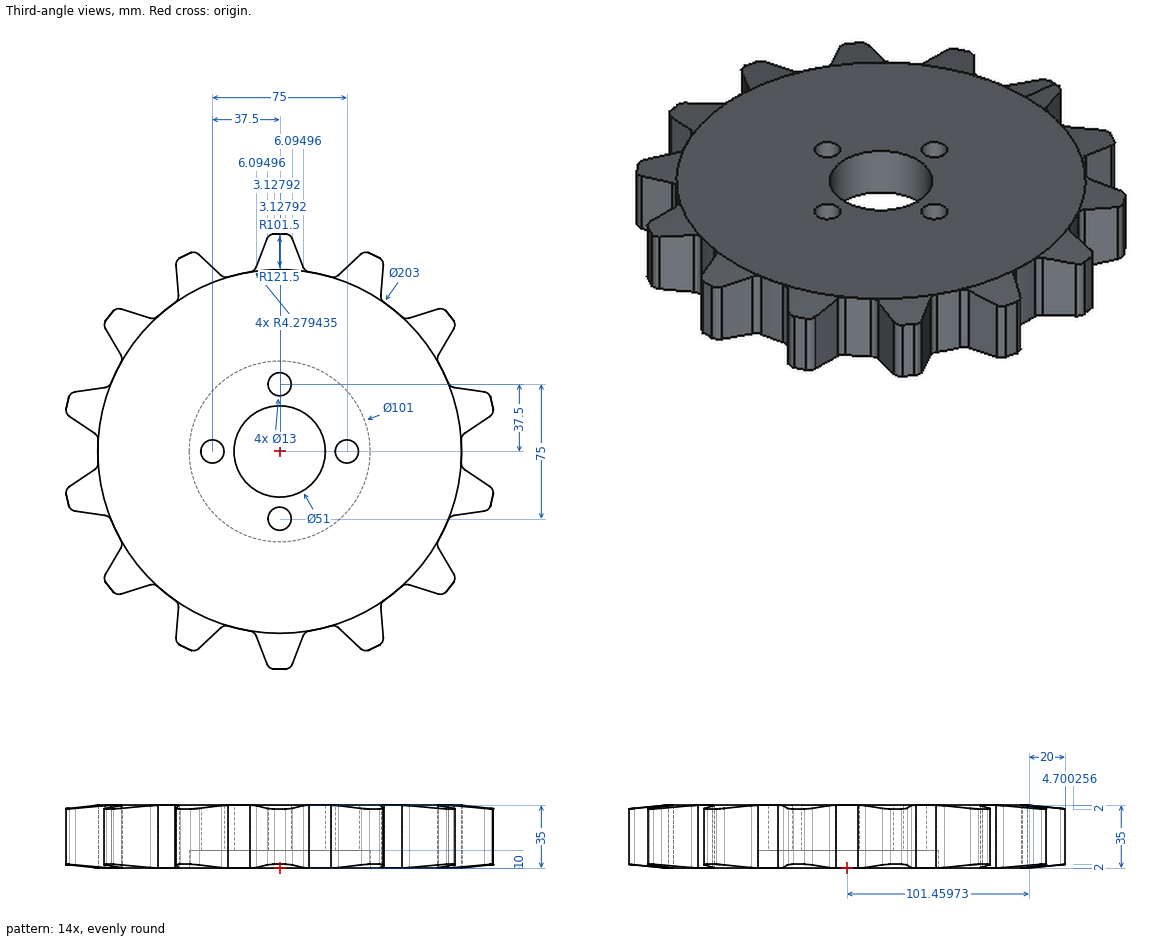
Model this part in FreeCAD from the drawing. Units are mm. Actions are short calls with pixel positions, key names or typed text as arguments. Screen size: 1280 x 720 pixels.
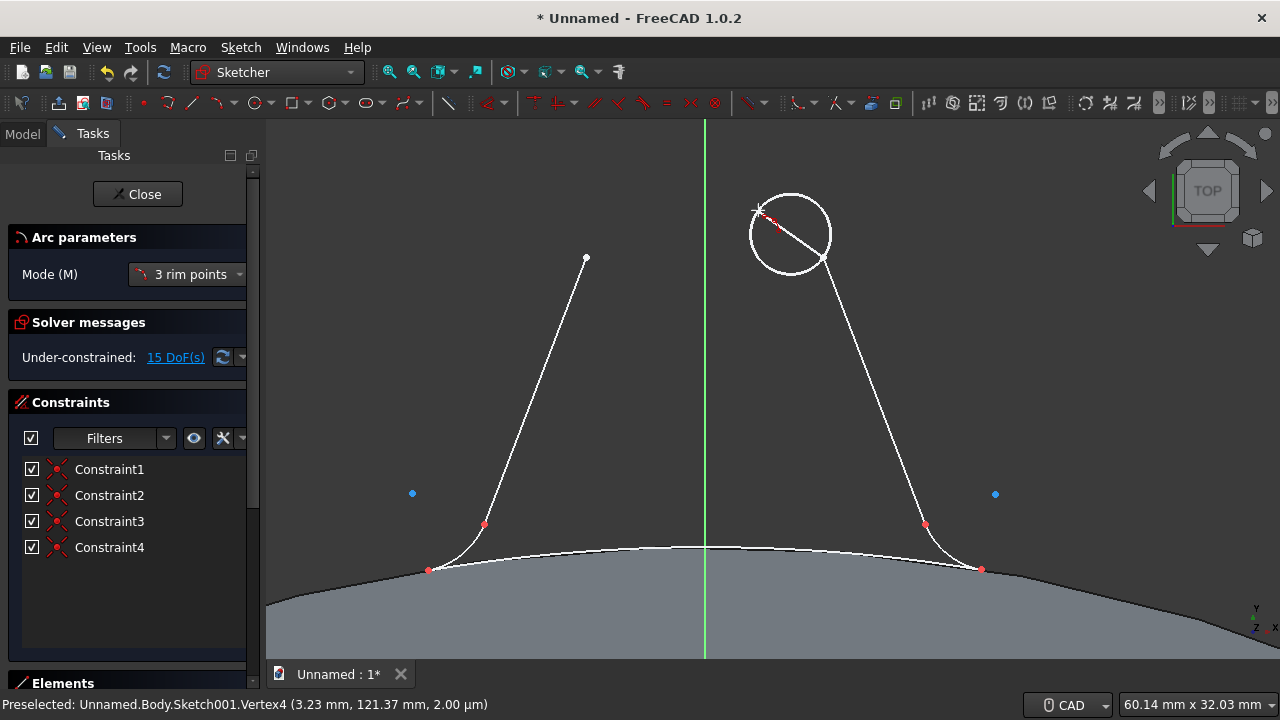
scroll(797, 223, up, 2)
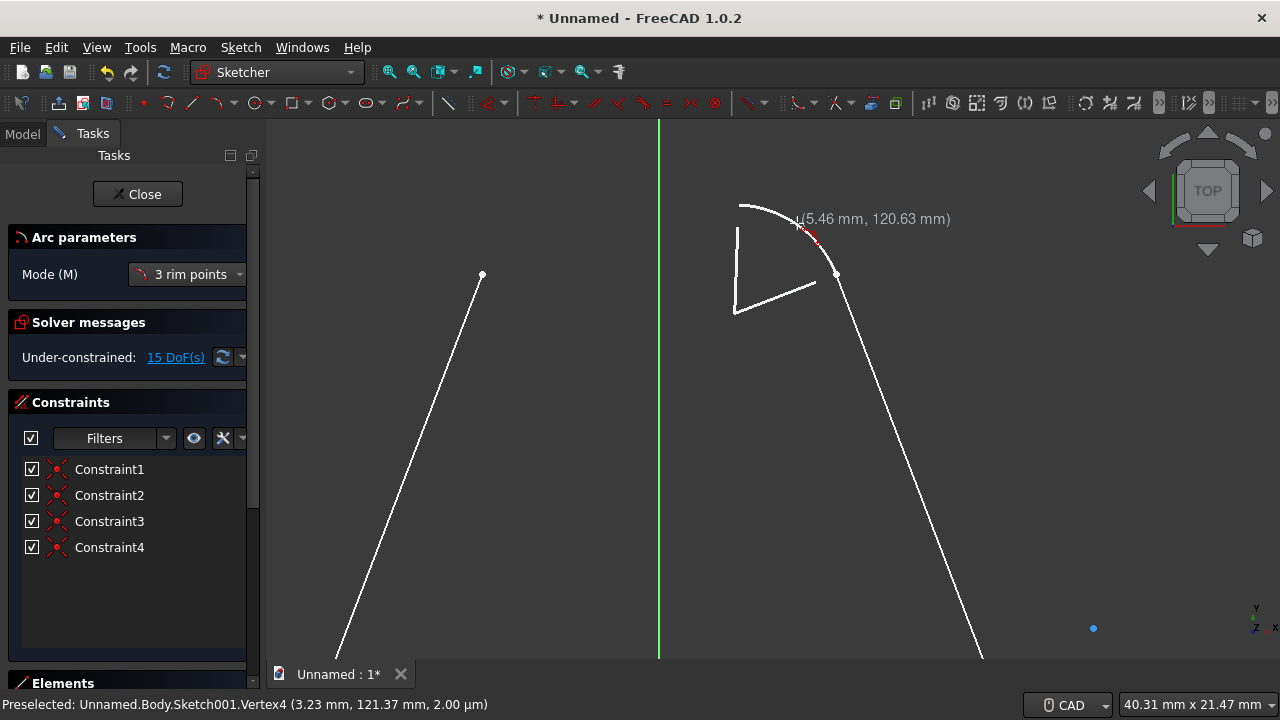
click(797, 223)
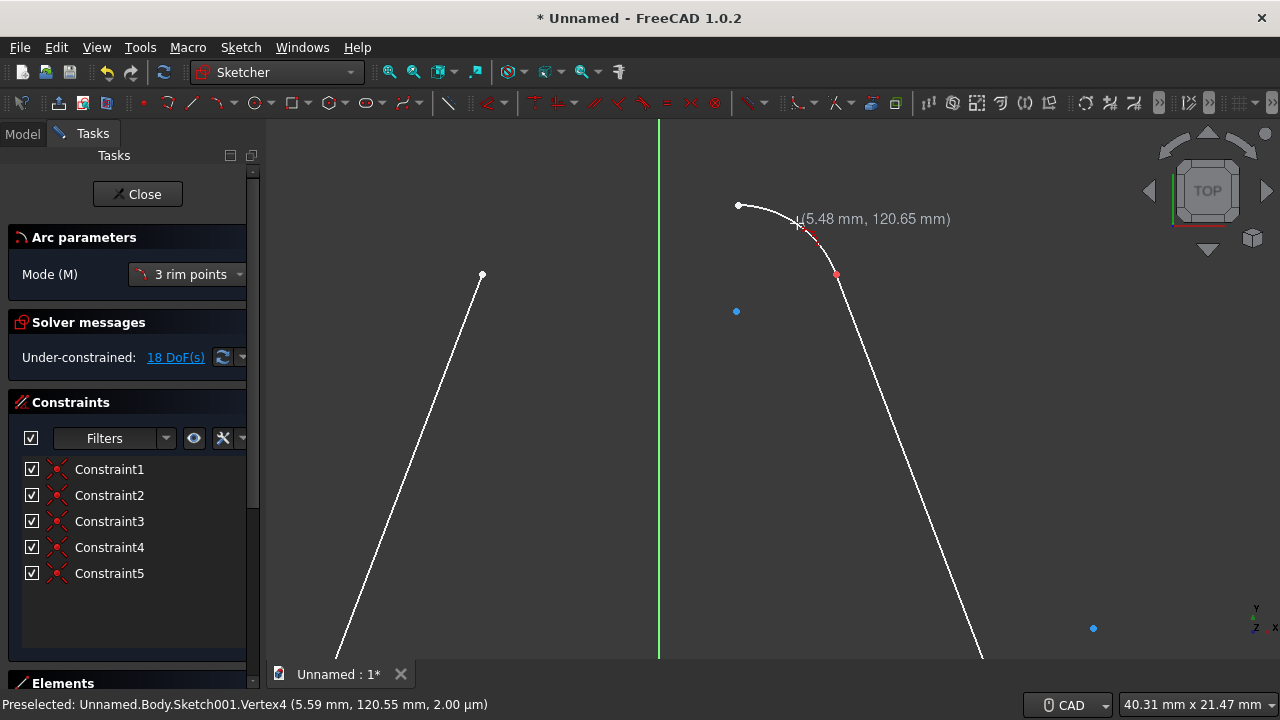
click(739, 205)
click(581, 204)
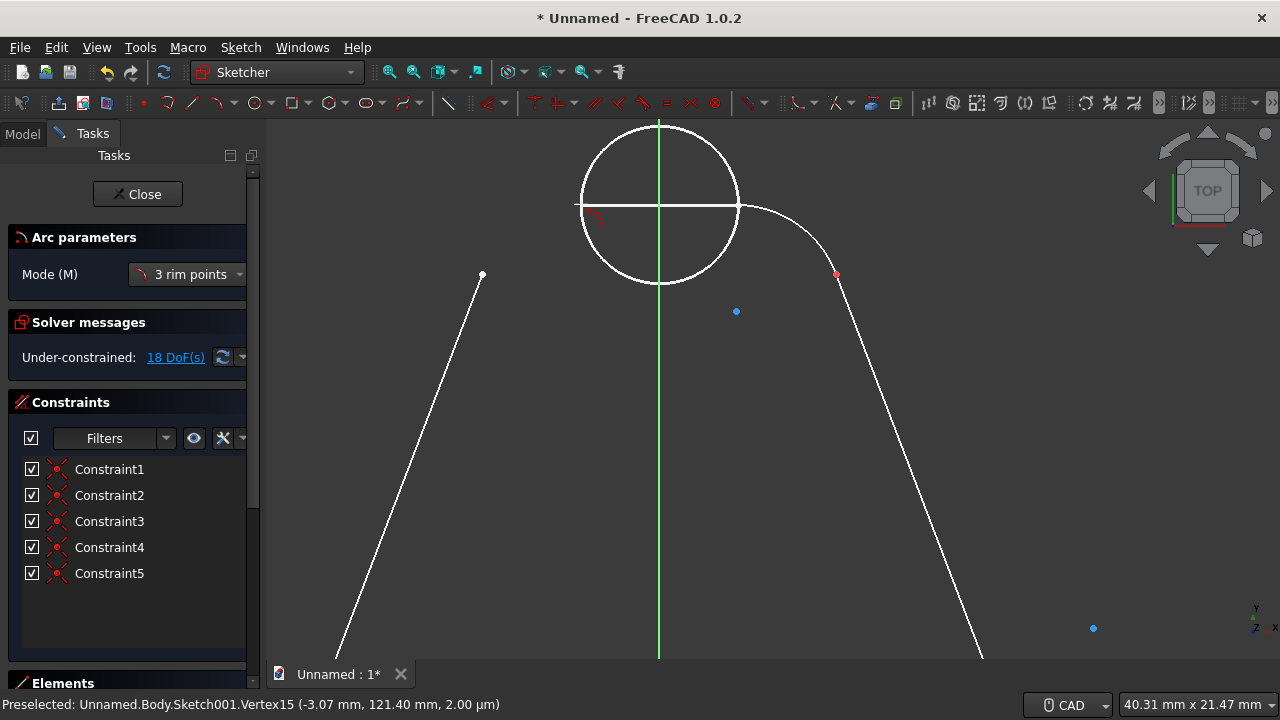
scroll(675, 203, up, 14)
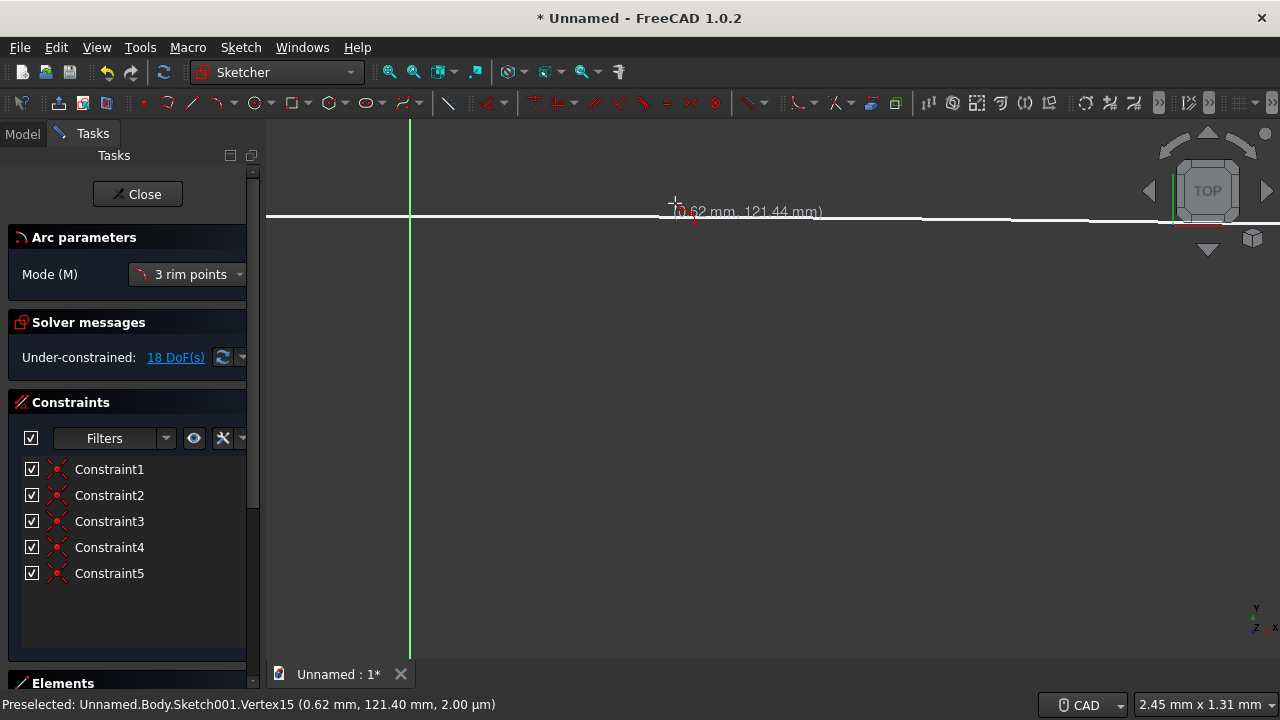
click(669, 194)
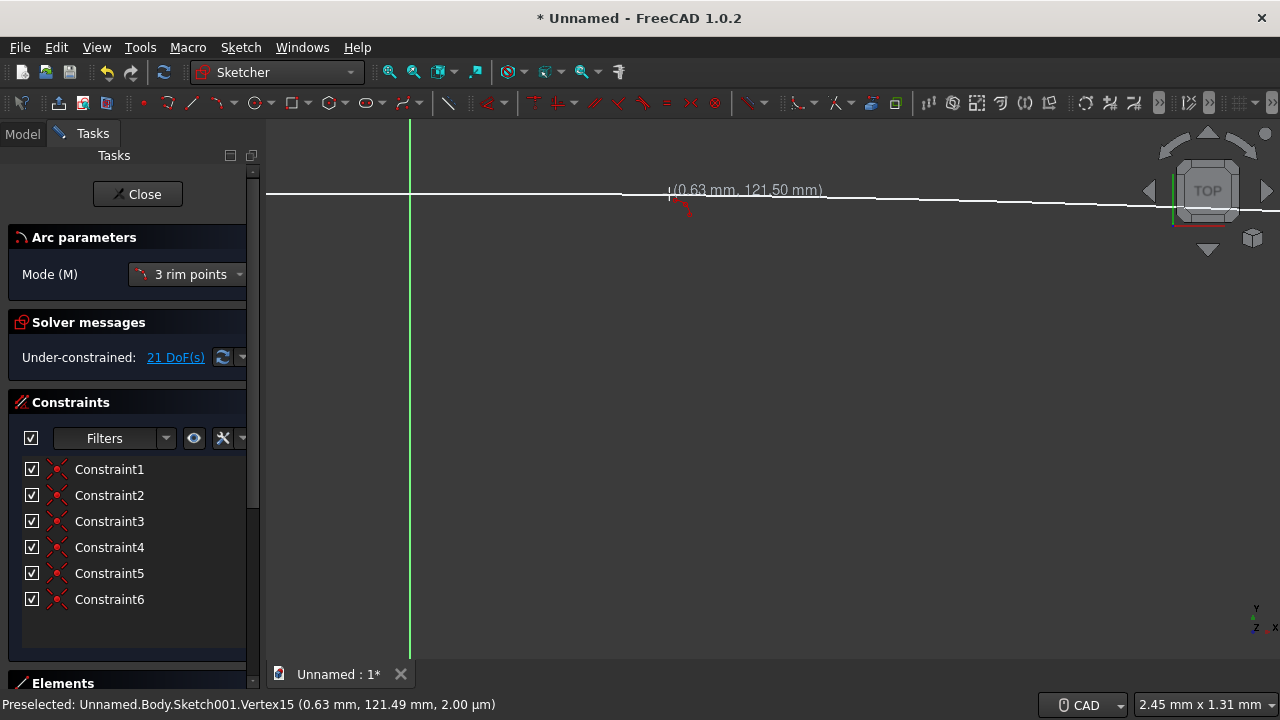
scroll(717, 210, down, 16)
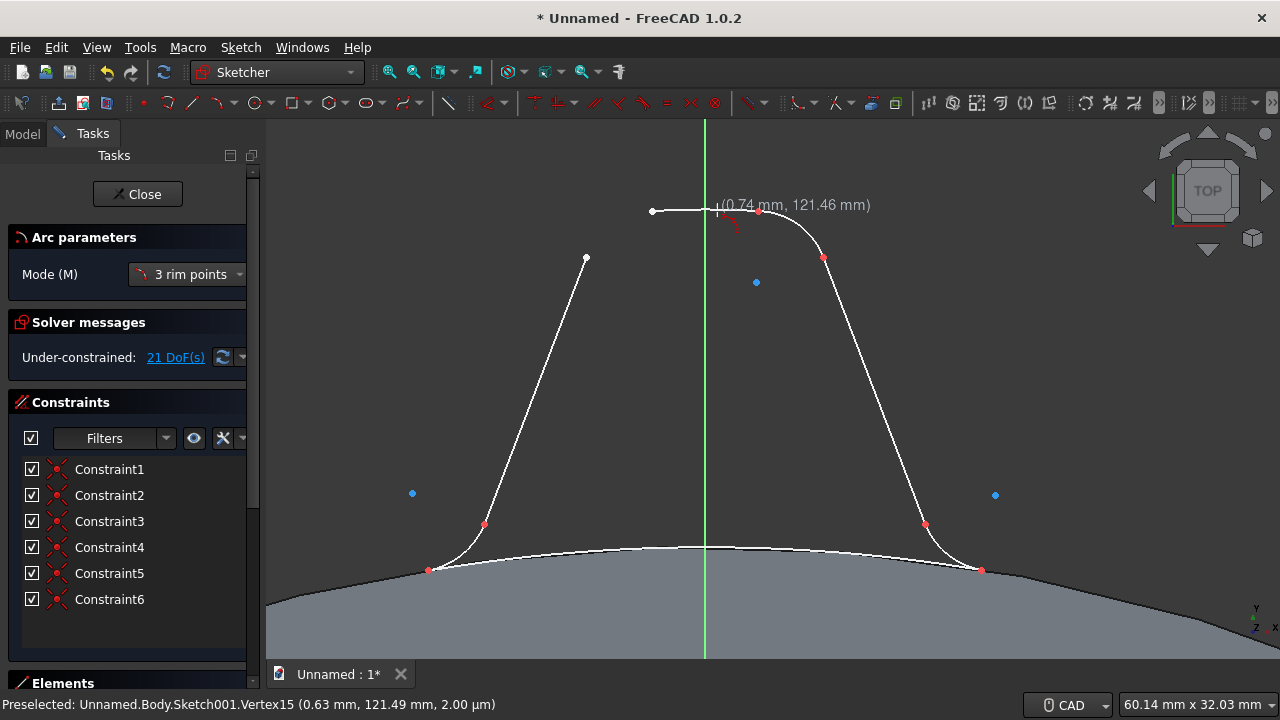
click(652, 211)
click(586, 258)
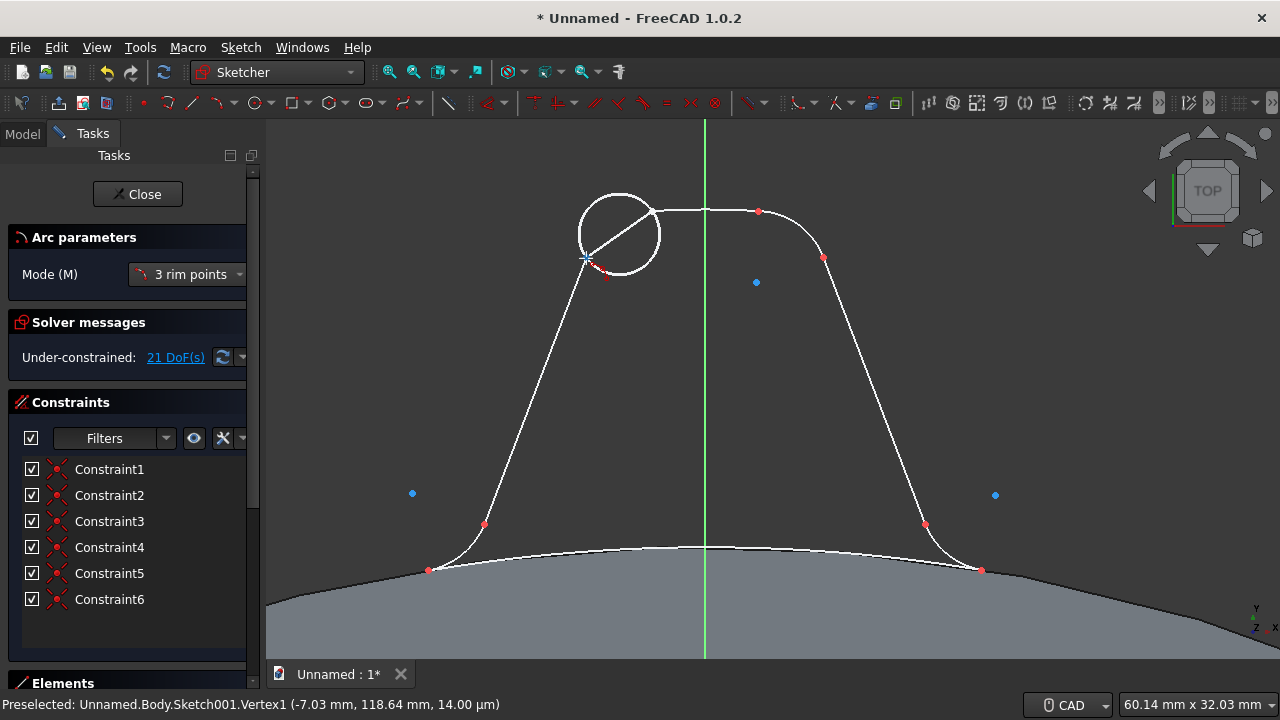
scroll(612, 223, up, 2)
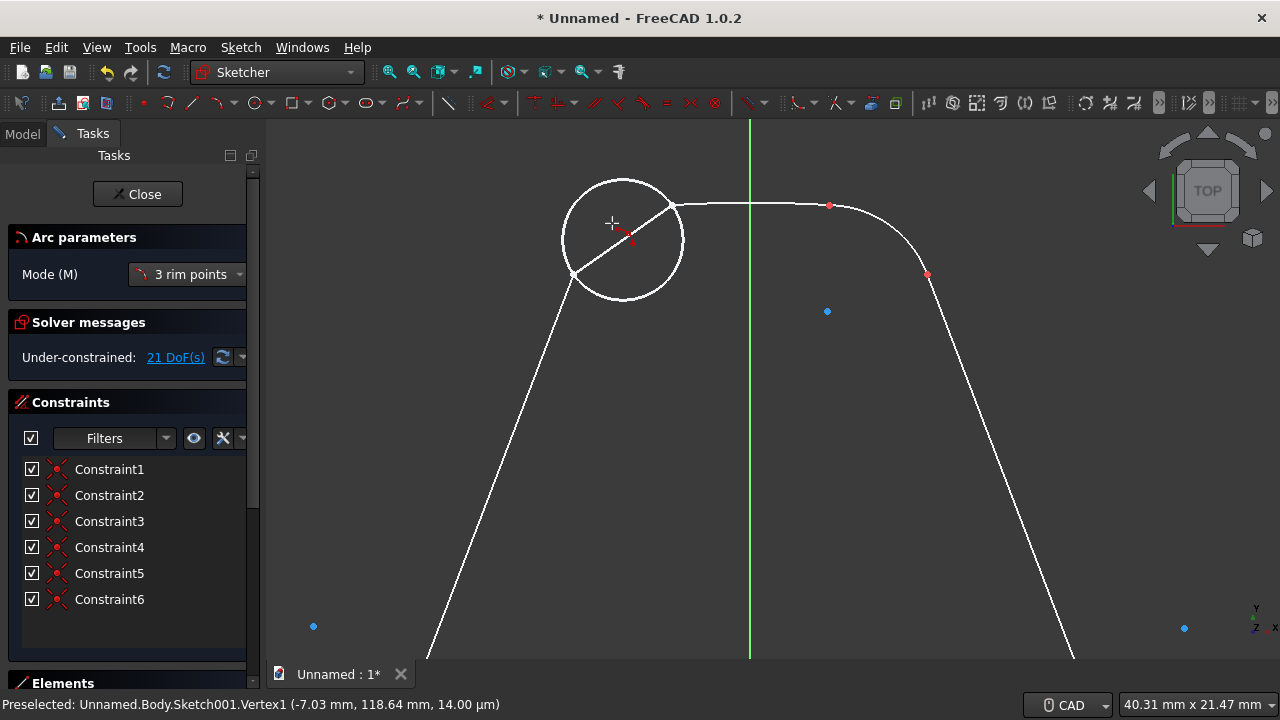
click(612, 223)
key(Escape)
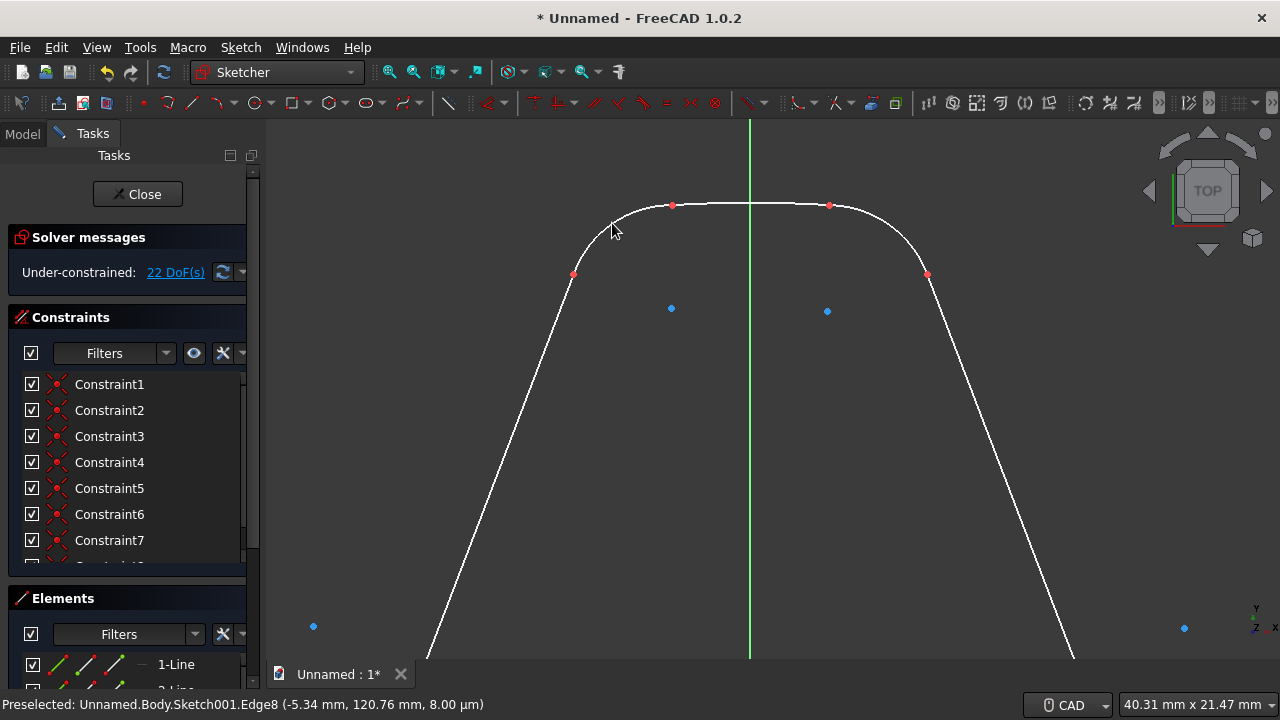
click(528, 394)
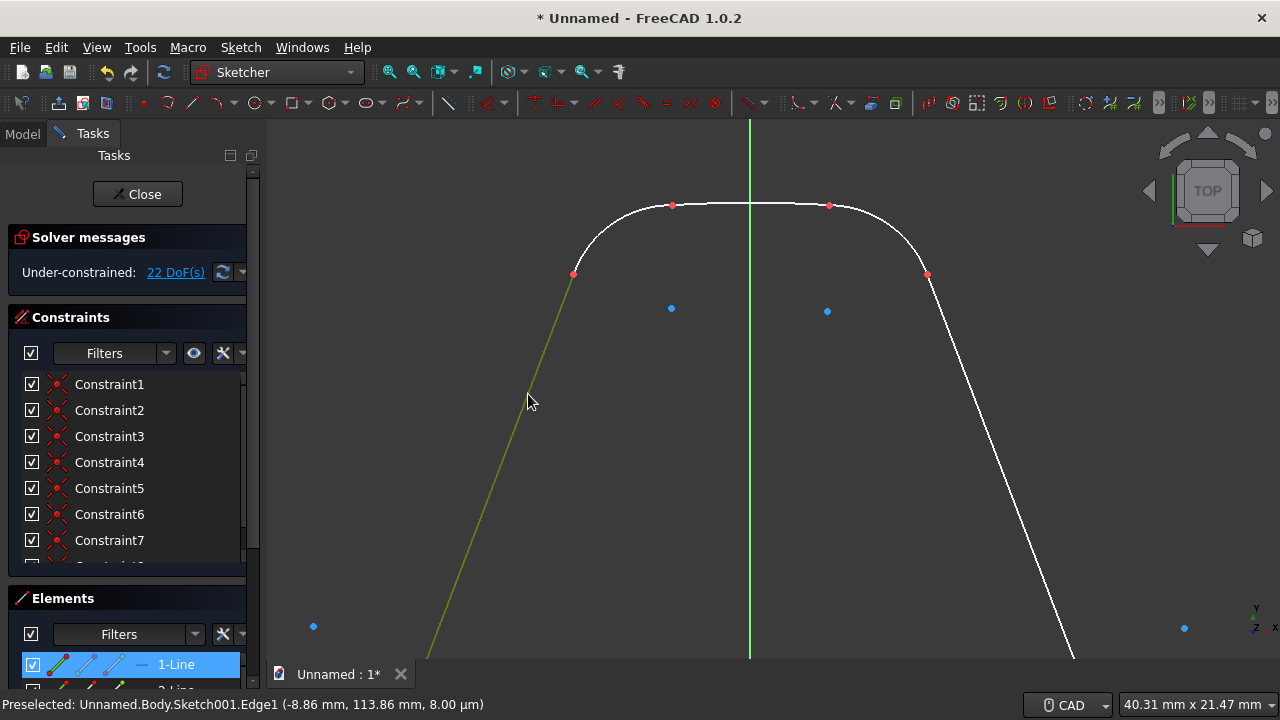
scroll(611, 222, down, 2)